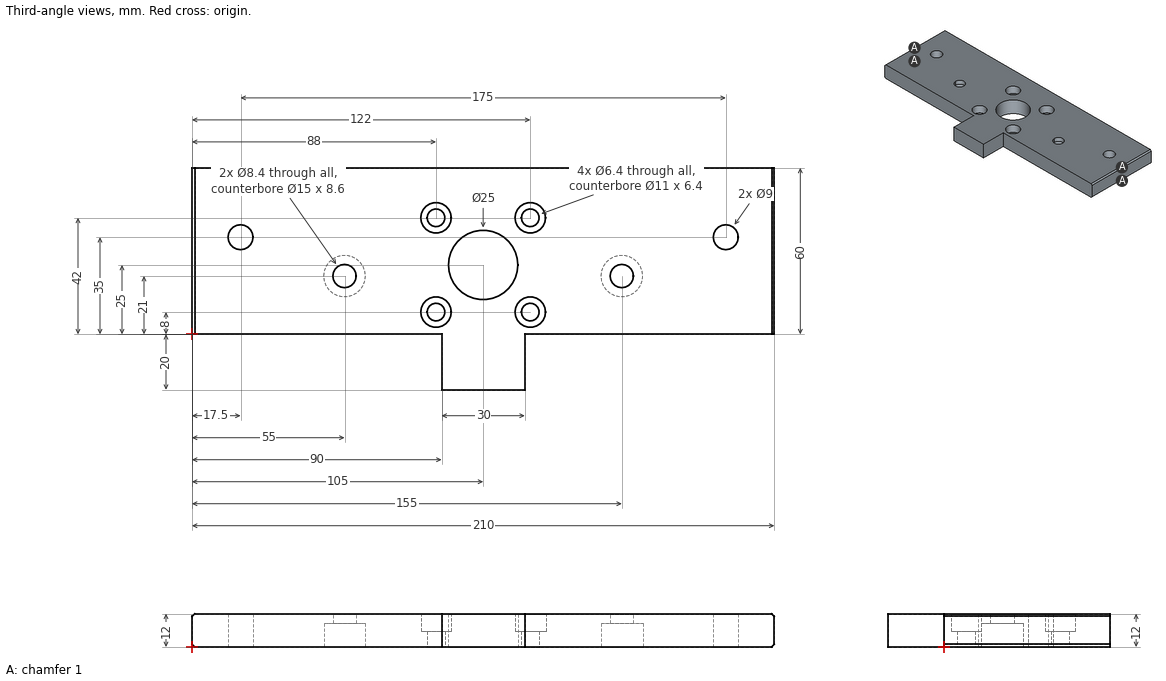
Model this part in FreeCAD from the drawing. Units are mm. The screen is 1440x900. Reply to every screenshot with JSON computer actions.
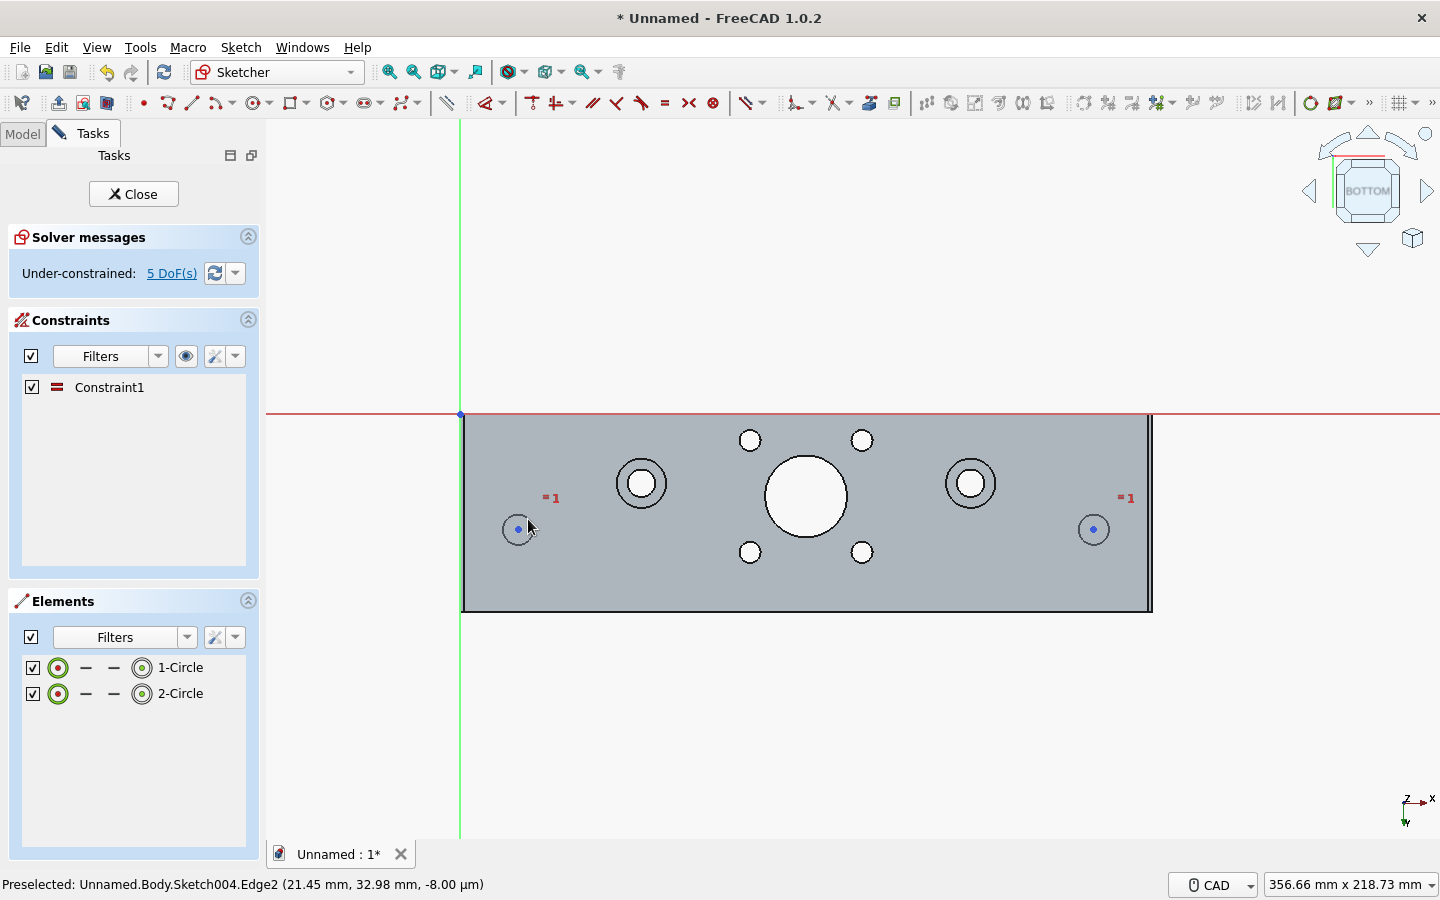
{"action": "left_click", "coordinate": [1094, 530]}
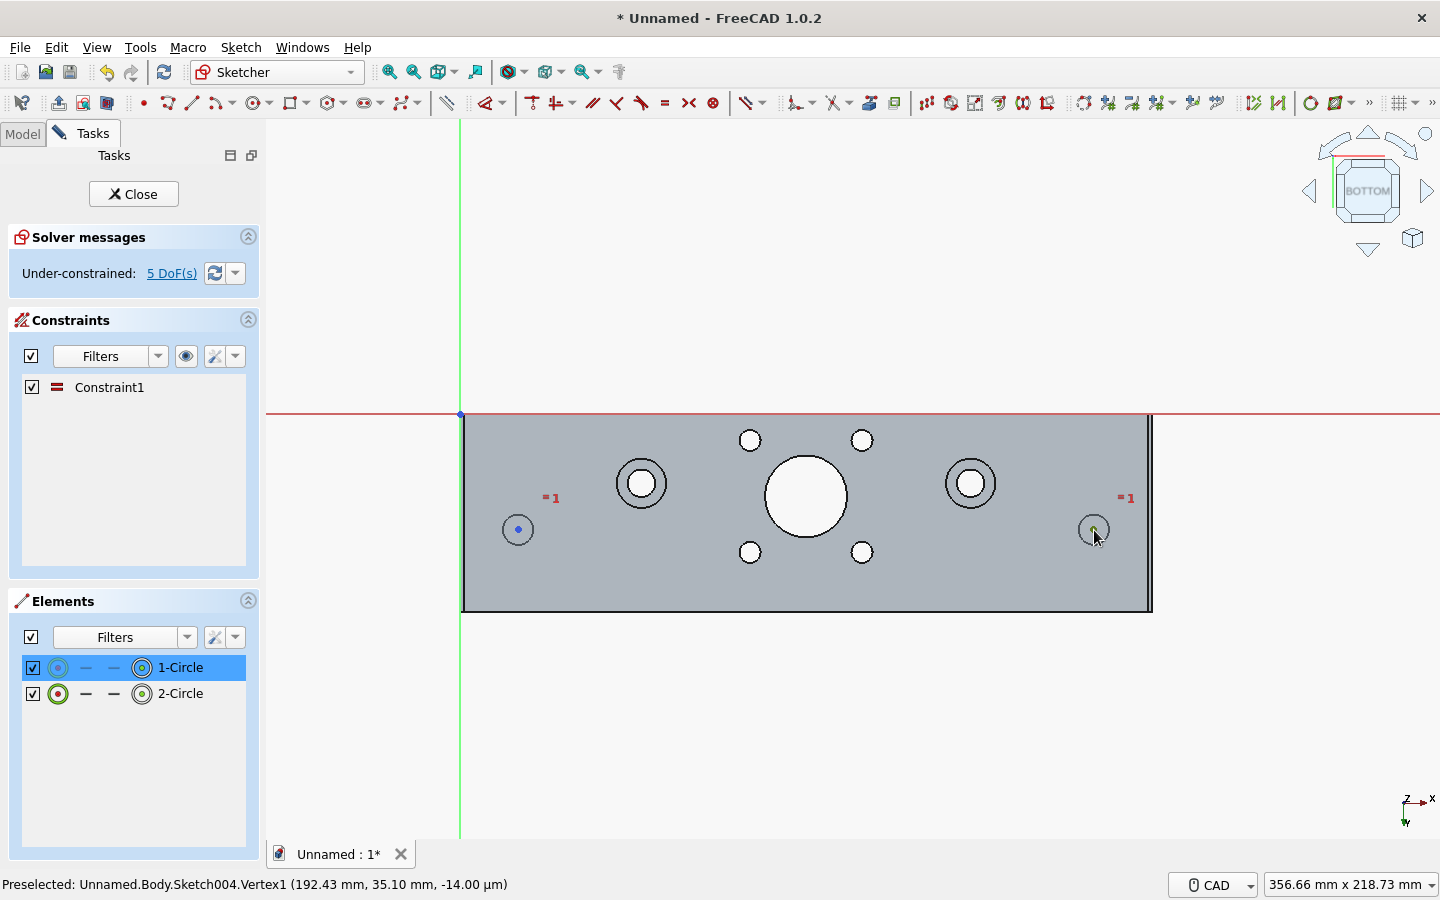
{"action": "left_click", "coordinate": [518, 530]}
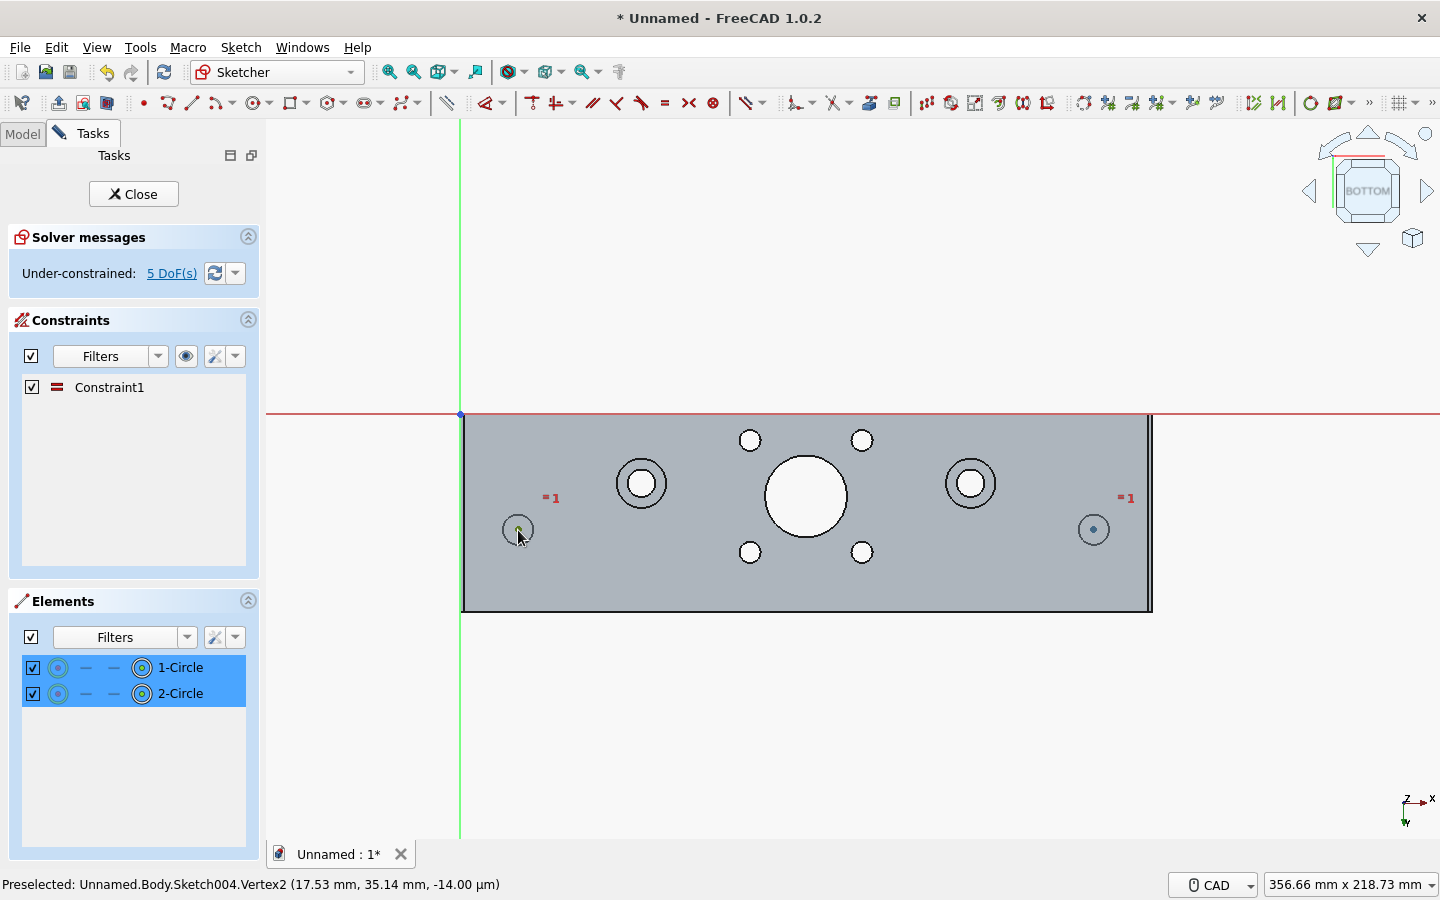
{"action": "key", "text": "h"}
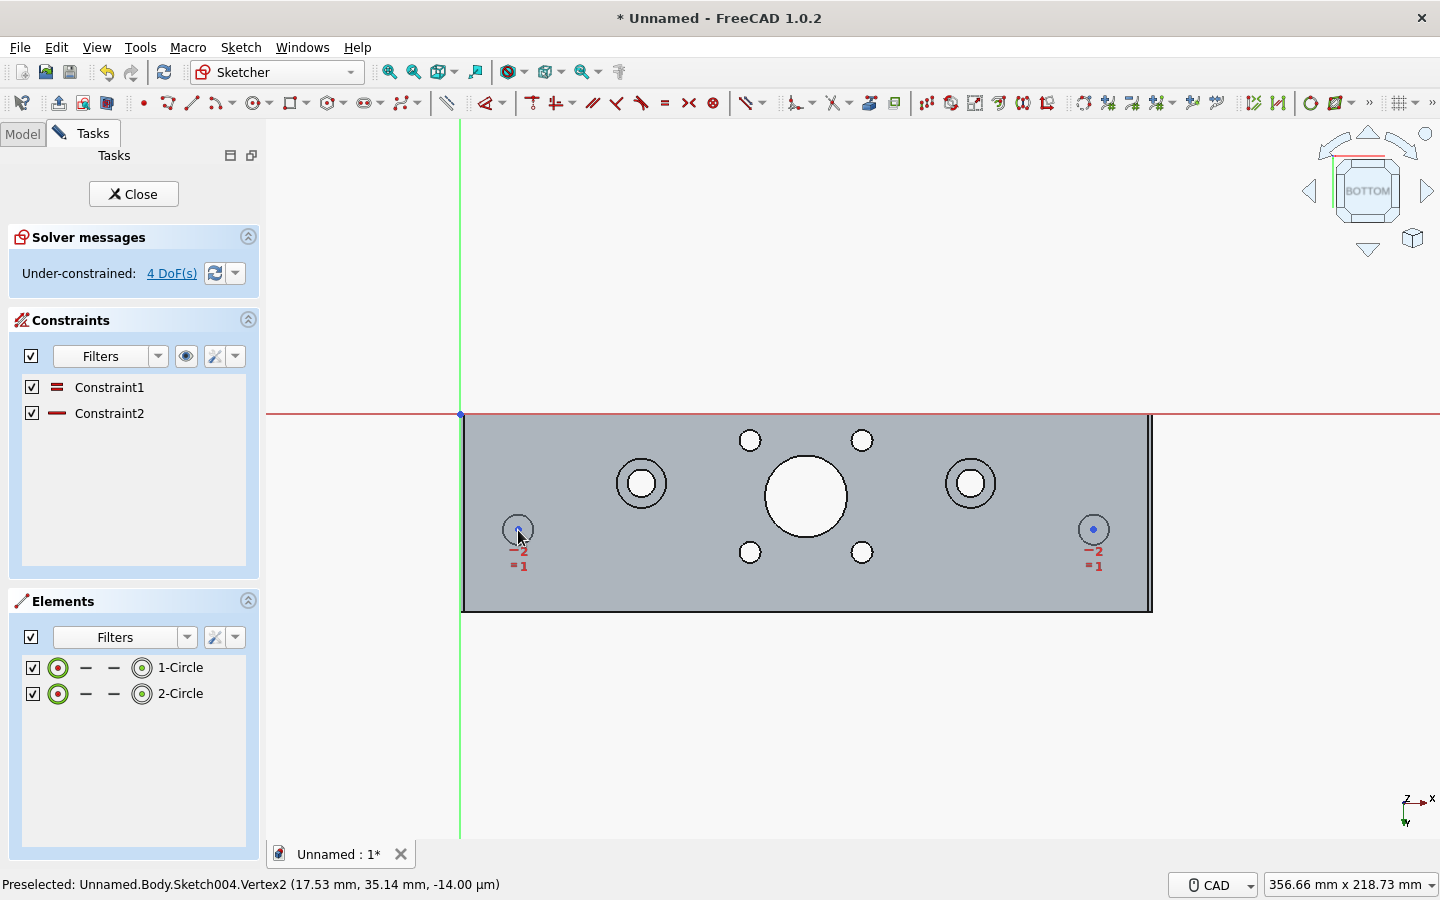
{"action": "key", "text": "d"}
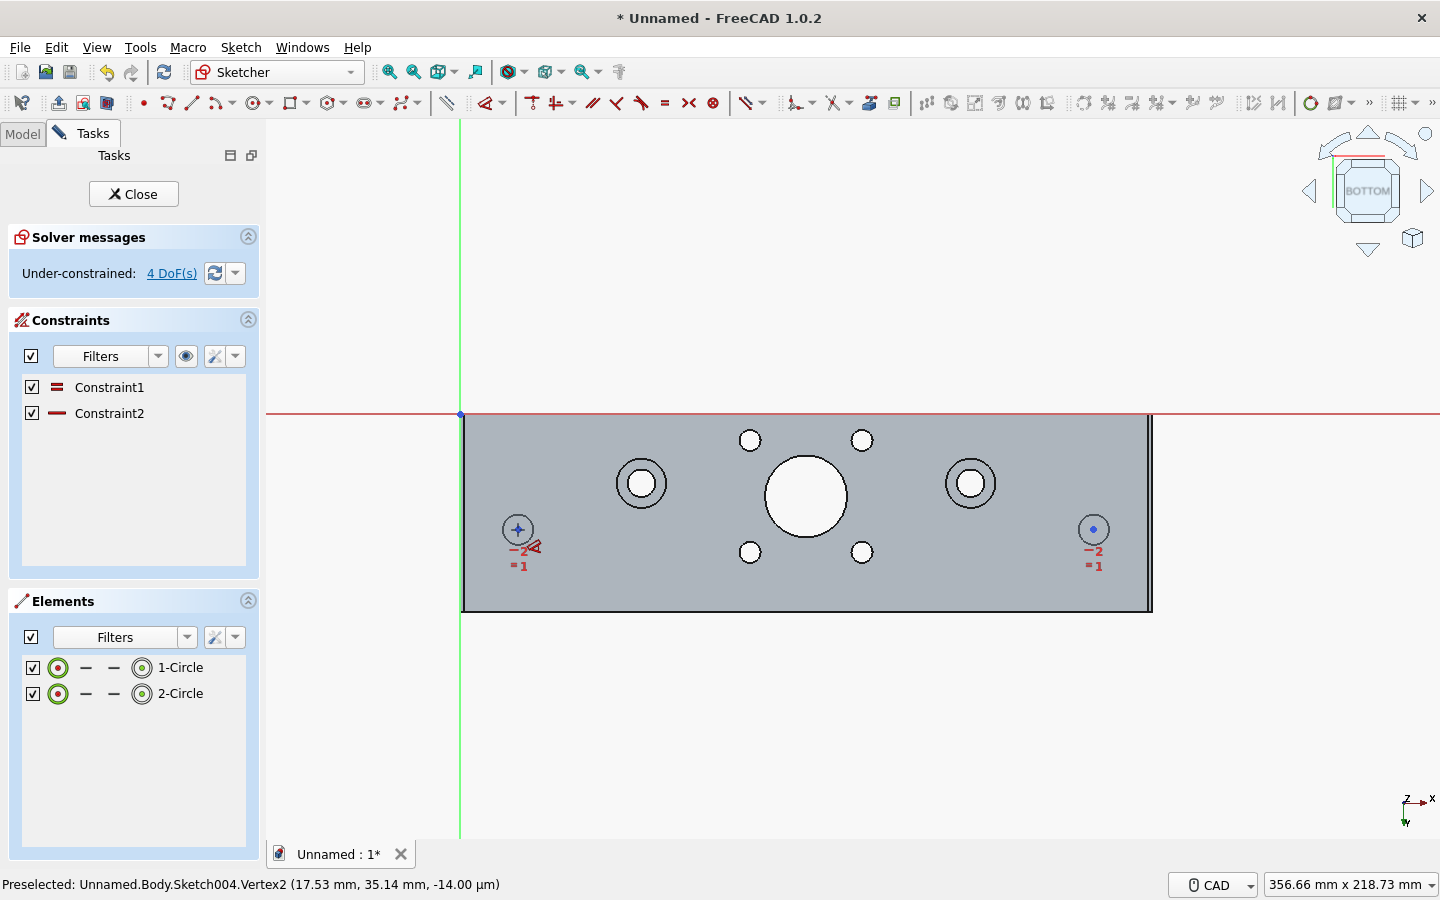
{"action": "scroll", "coordinate": [1104, 519], "scroll_direction": "up", "scroll_amount": 2}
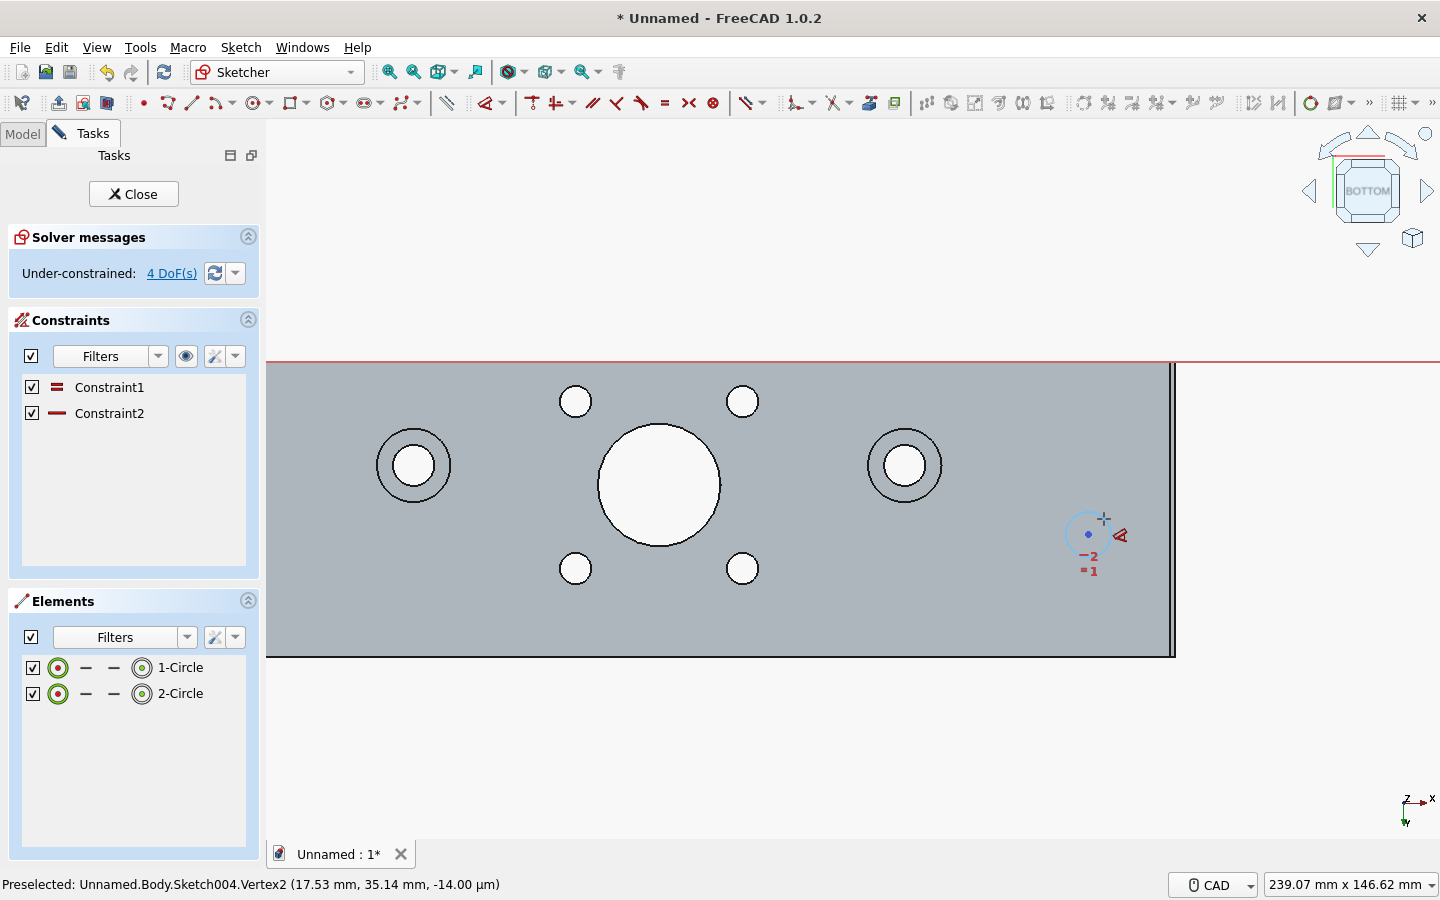
{"action": "left_click", "coordinate": [1104, 519]}
{"action": "left_click", "coordinate": [1127, 496]}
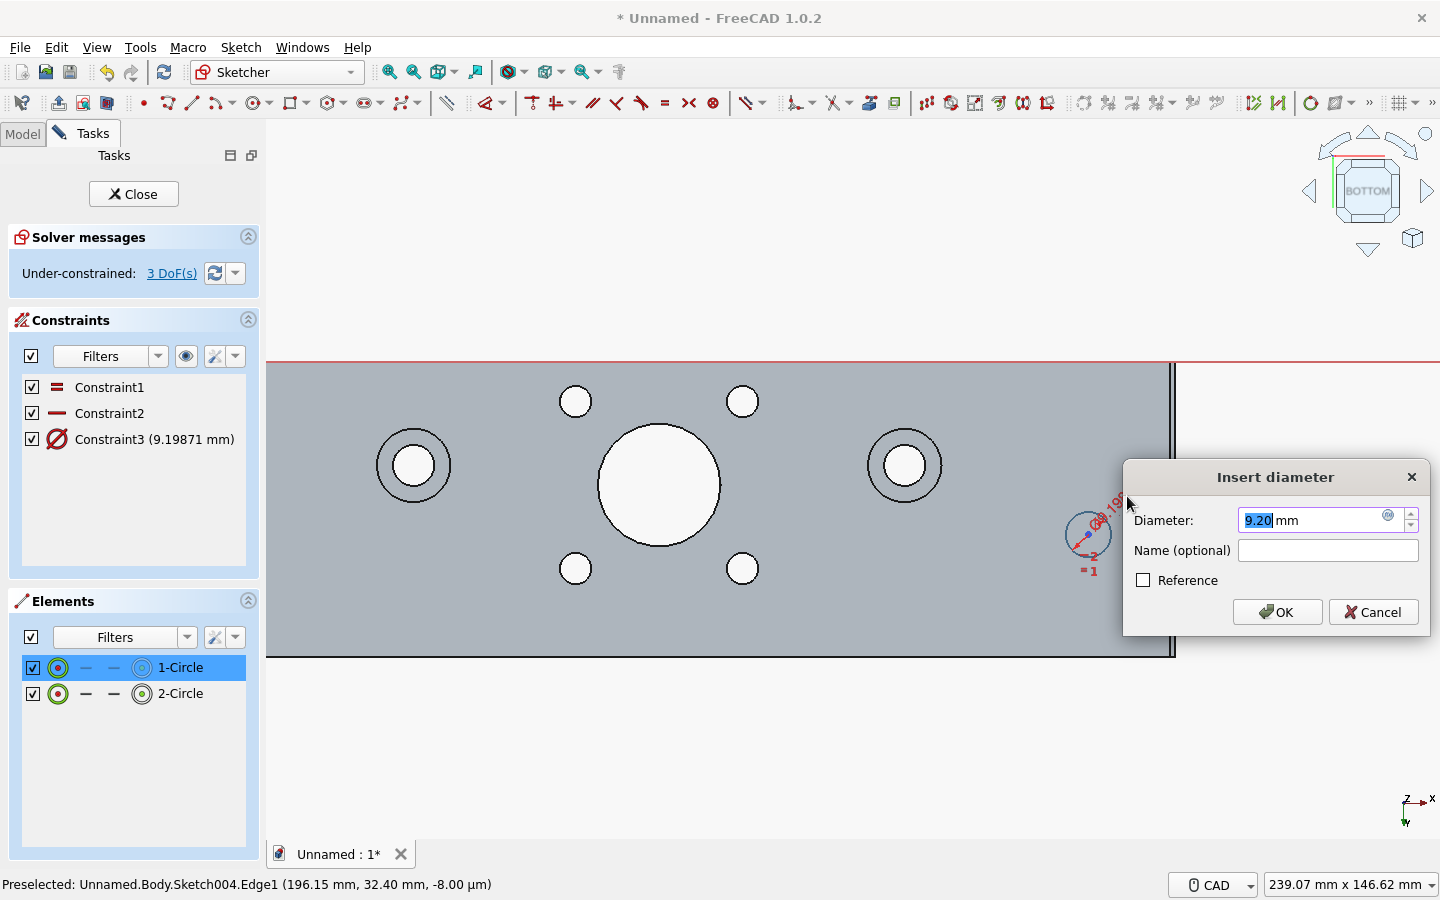
{"action": "type", "text": "9"}
{"action": "key", "text": "Return"}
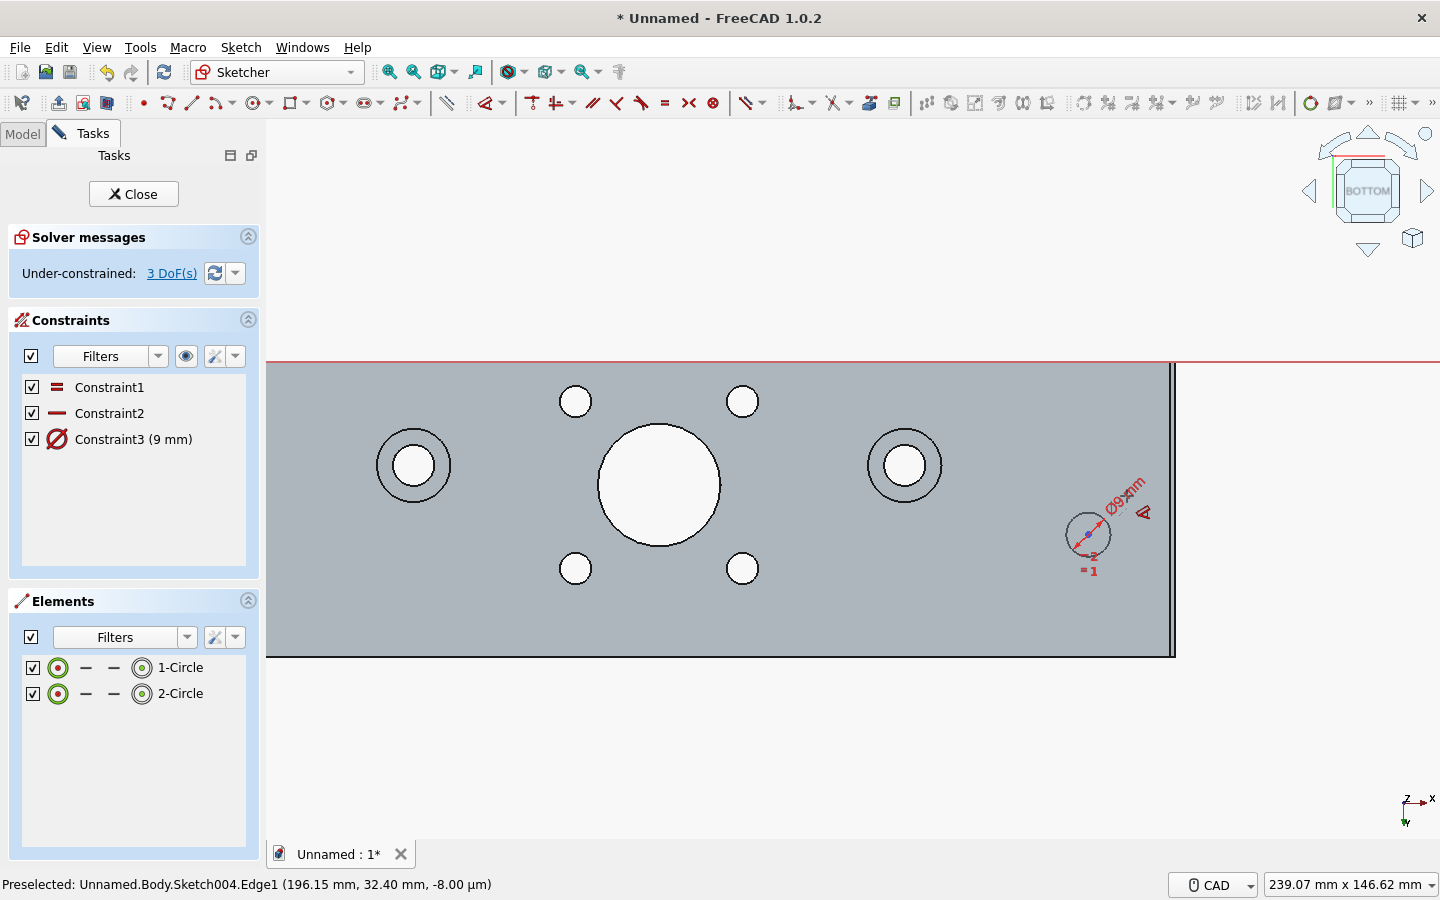
{"action": "left_click", "coordinate": [1088, 535]}
{"action": "left_click", "coordinate": [1122, 448]}